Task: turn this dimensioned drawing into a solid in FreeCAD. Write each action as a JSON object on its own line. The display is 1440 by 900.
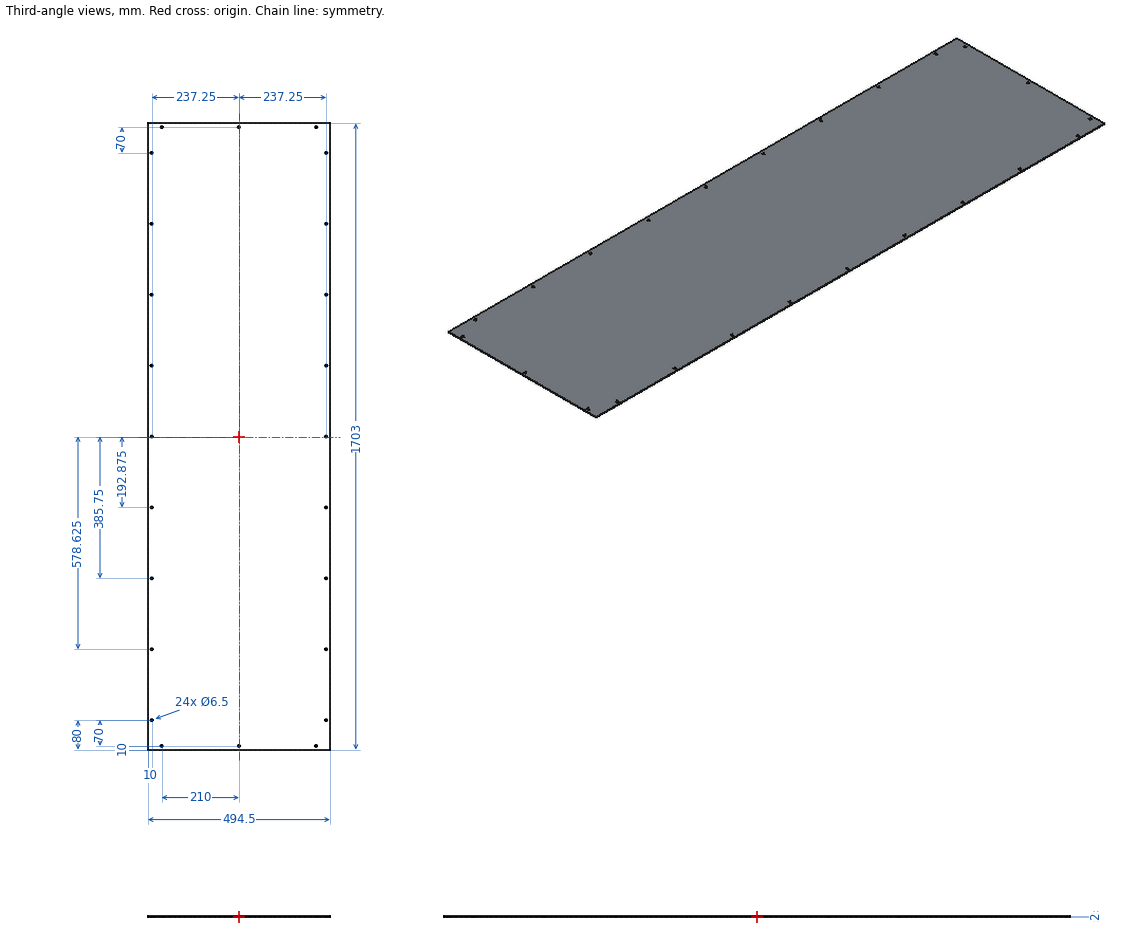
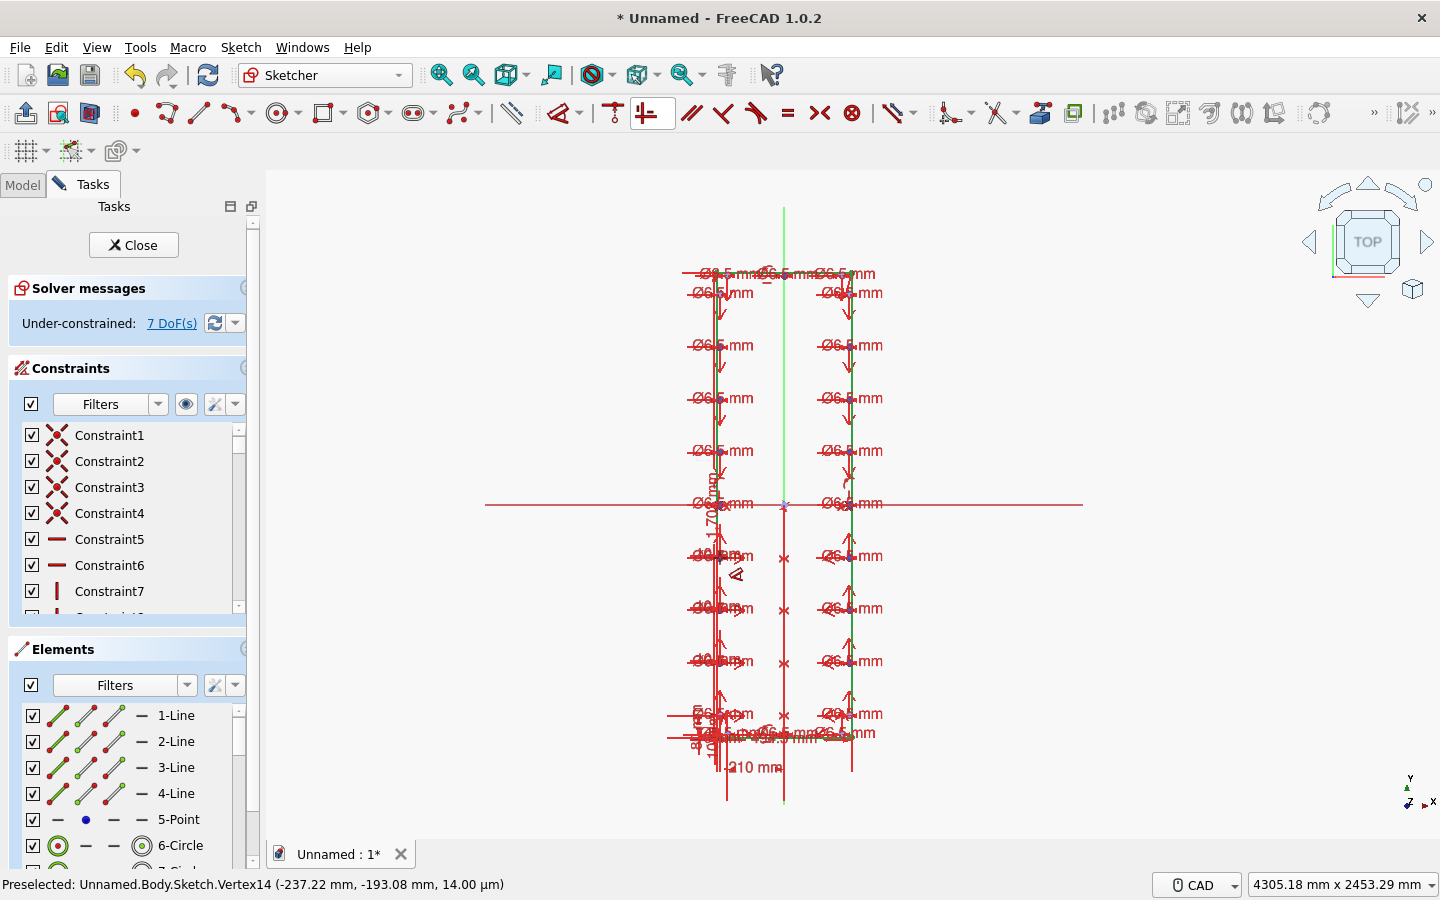
{"action": "scroll", "coordinate": [720, 716], "scroll_direction": "up", "scroll_amount": 4}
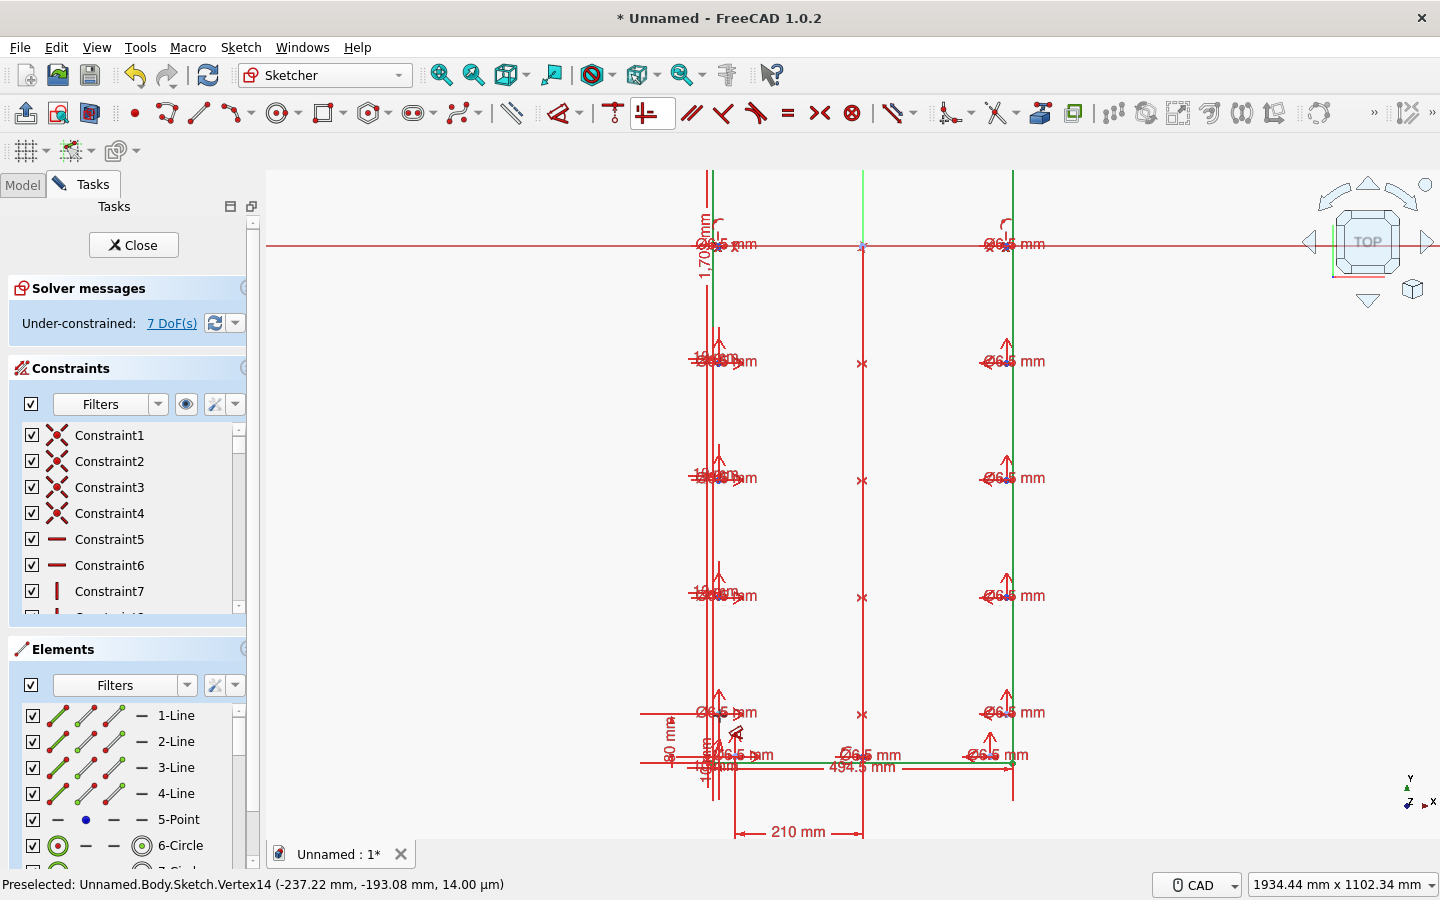
{"action": "left_click", "coordinate": [719, 714]}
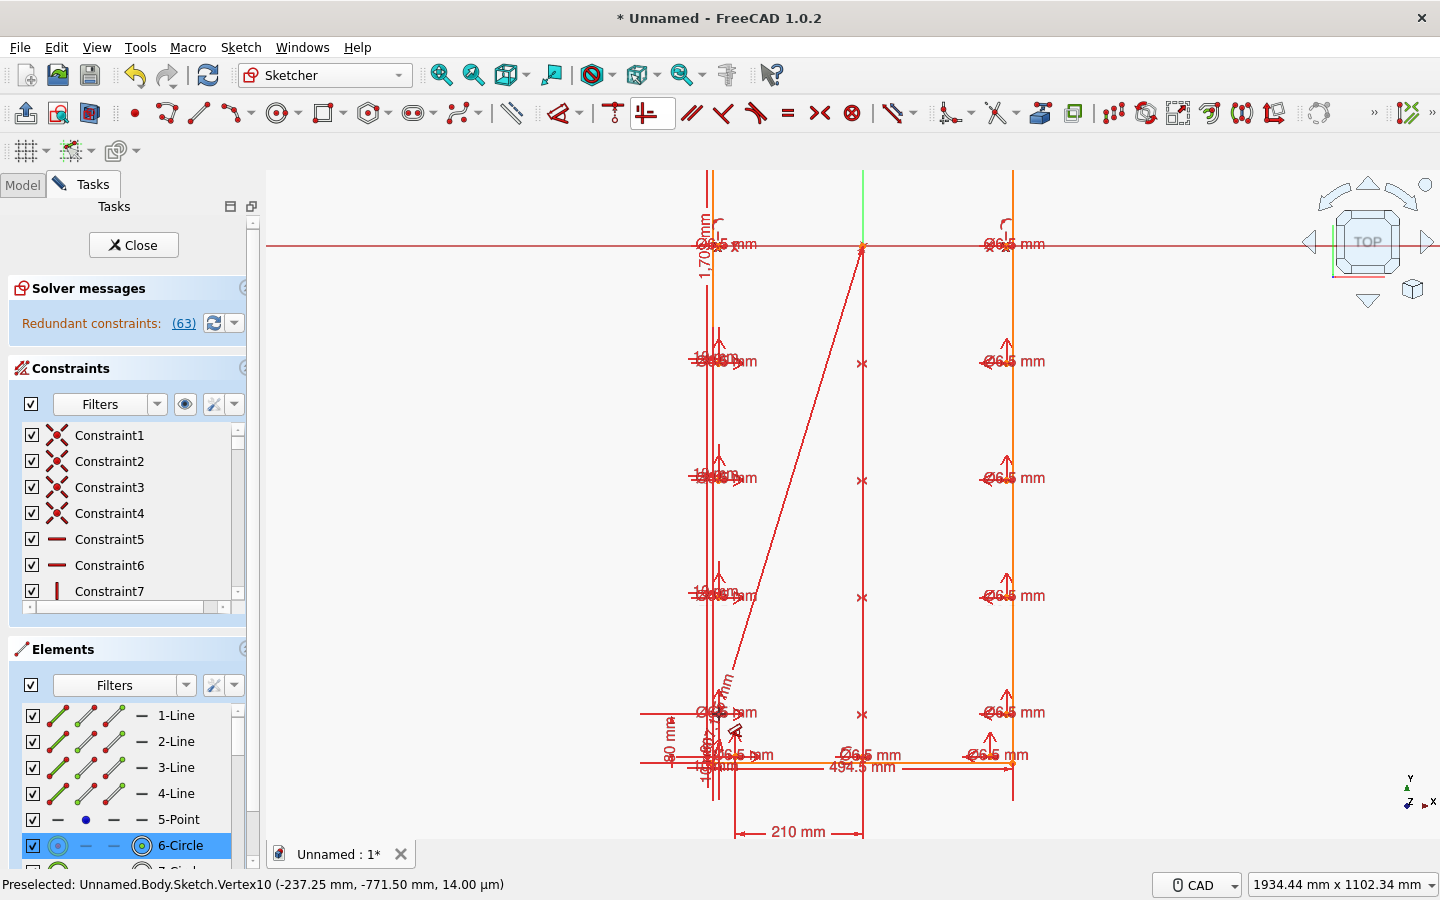
{"action": "left_click", "coordinate": [863, 757]}
{"action": "left_click", "coordinate": [897, 736]}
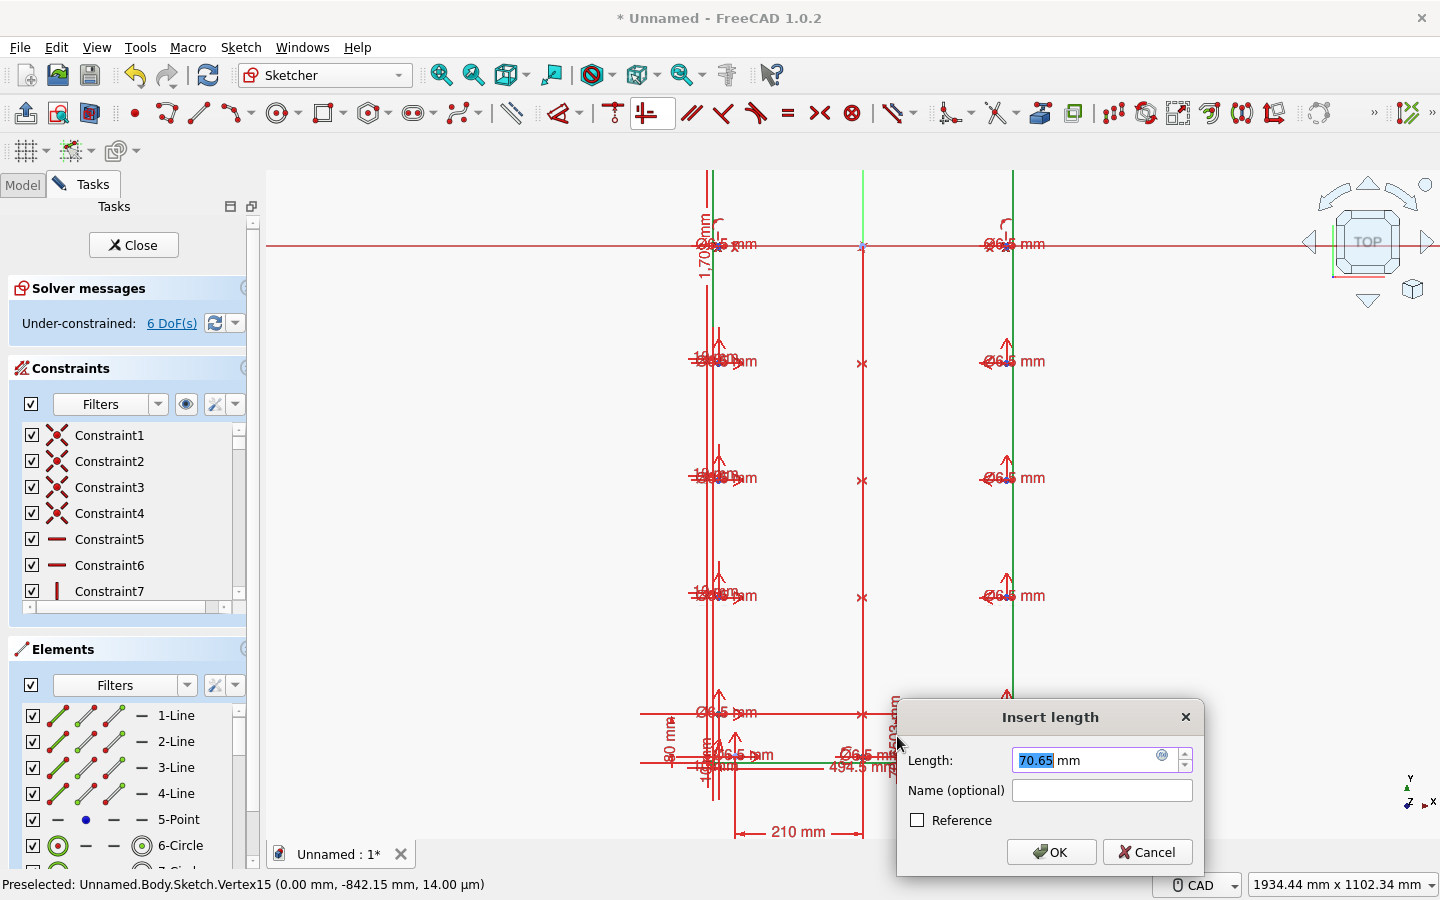
{"action": "type", "text": "70"}
{"action": "key", "text": "Return"}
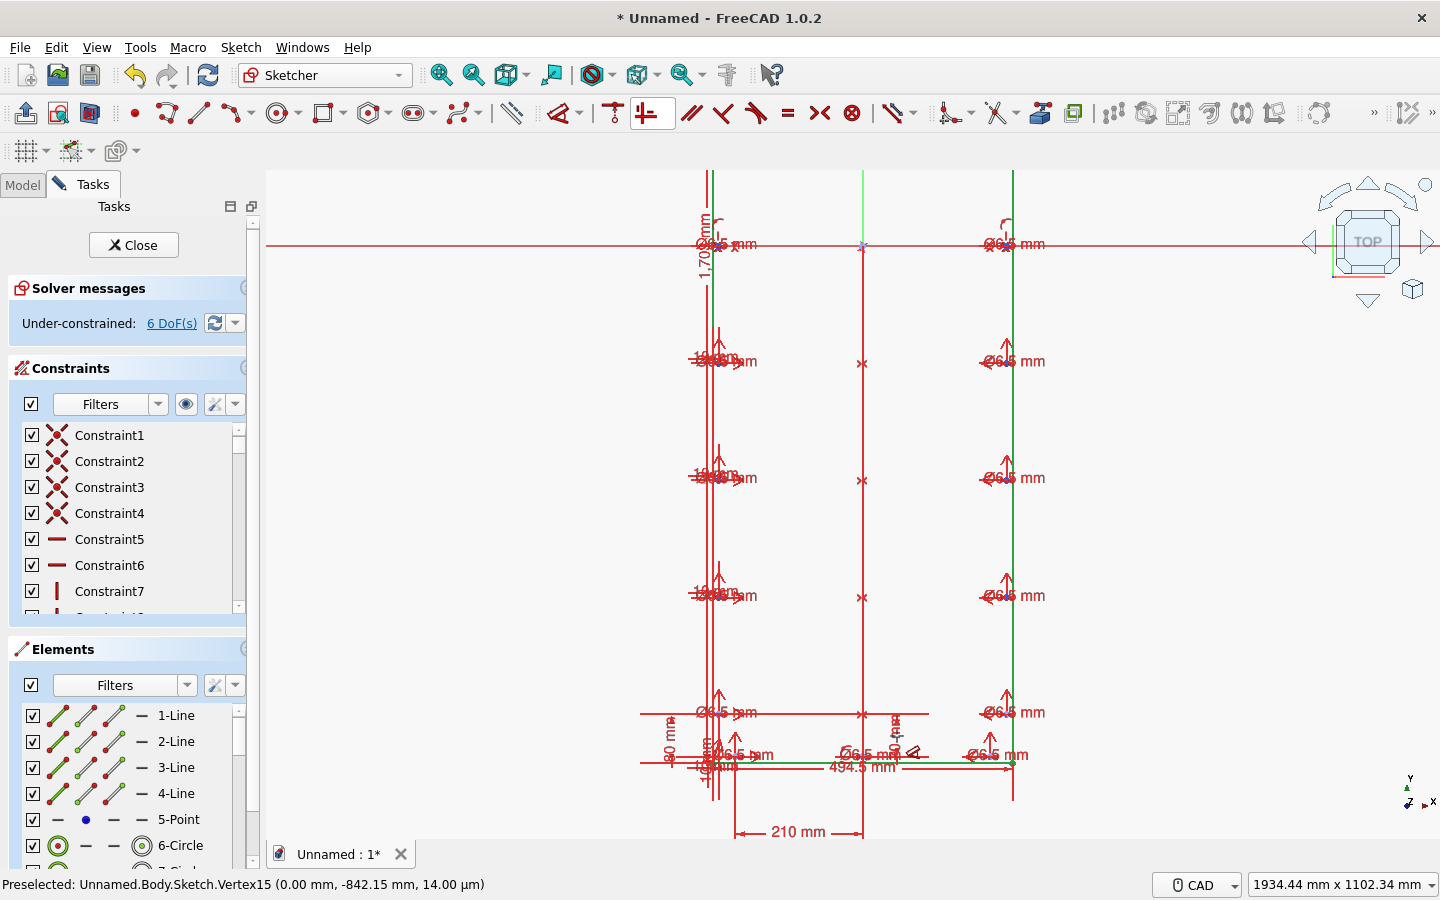
{"action": "scroll", "coordinate": [721, 715], "scroll_direction": "down", "scroll_amount": 4}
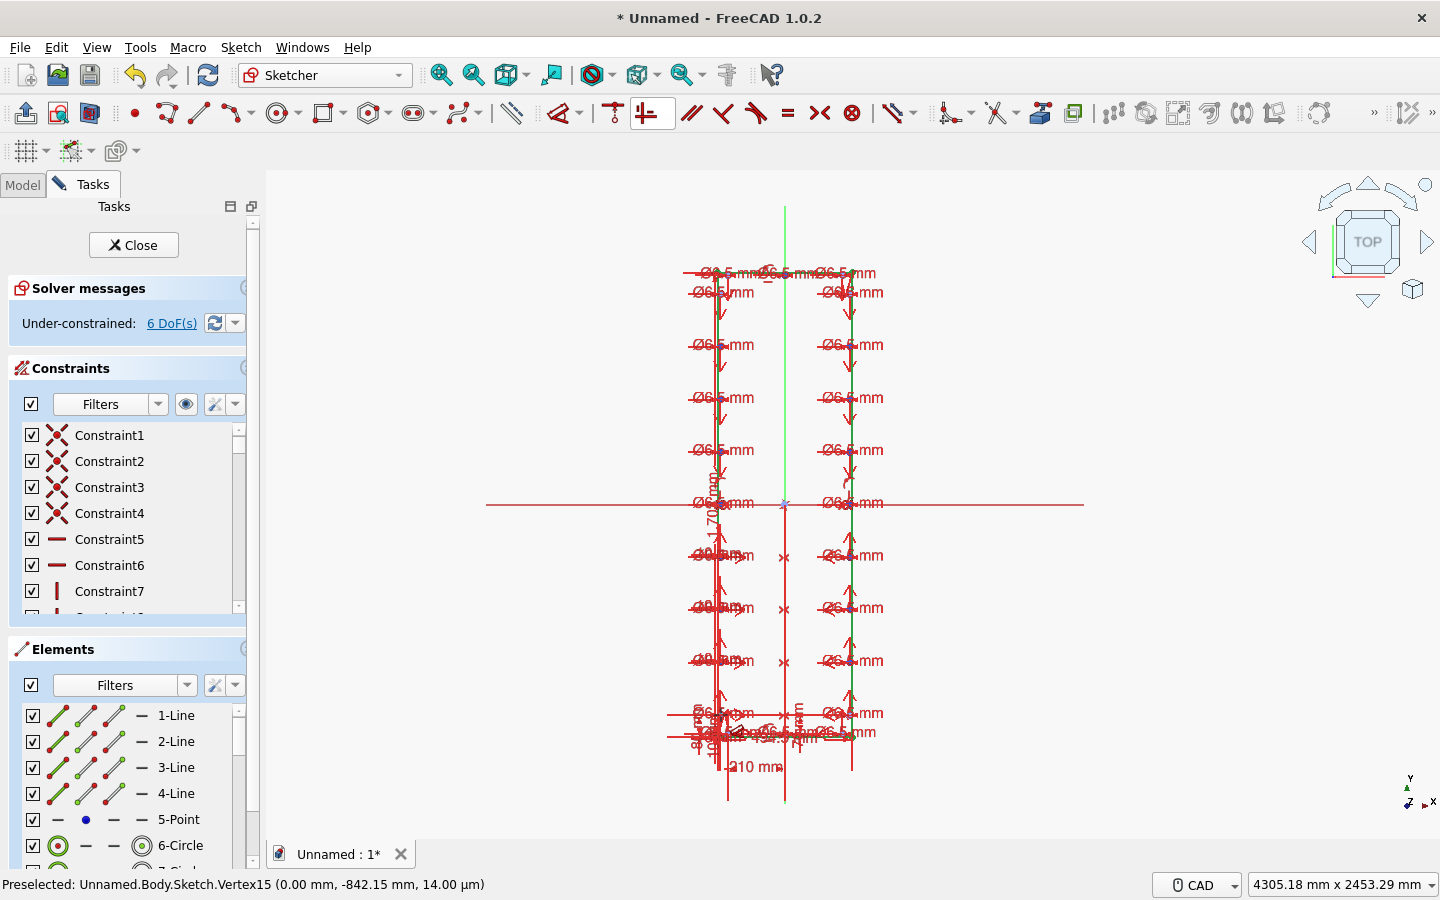
{"action": "scroll", "coordinate": [720, 294], "scroll_direction": "up", "scroll_amount": 4}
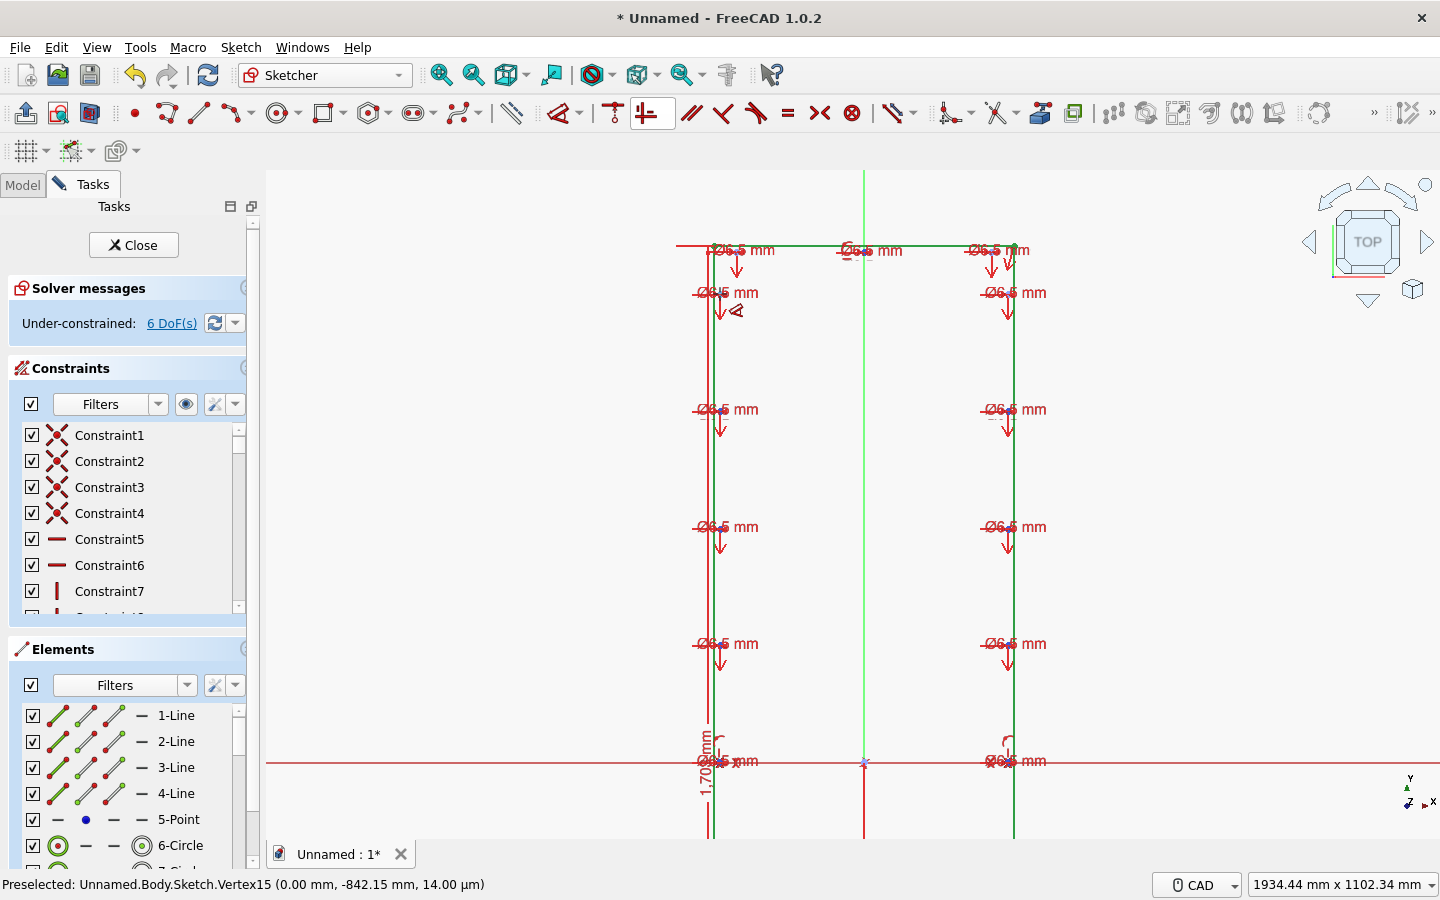
{"action": "left_click", "coordinate": [720, 295]}